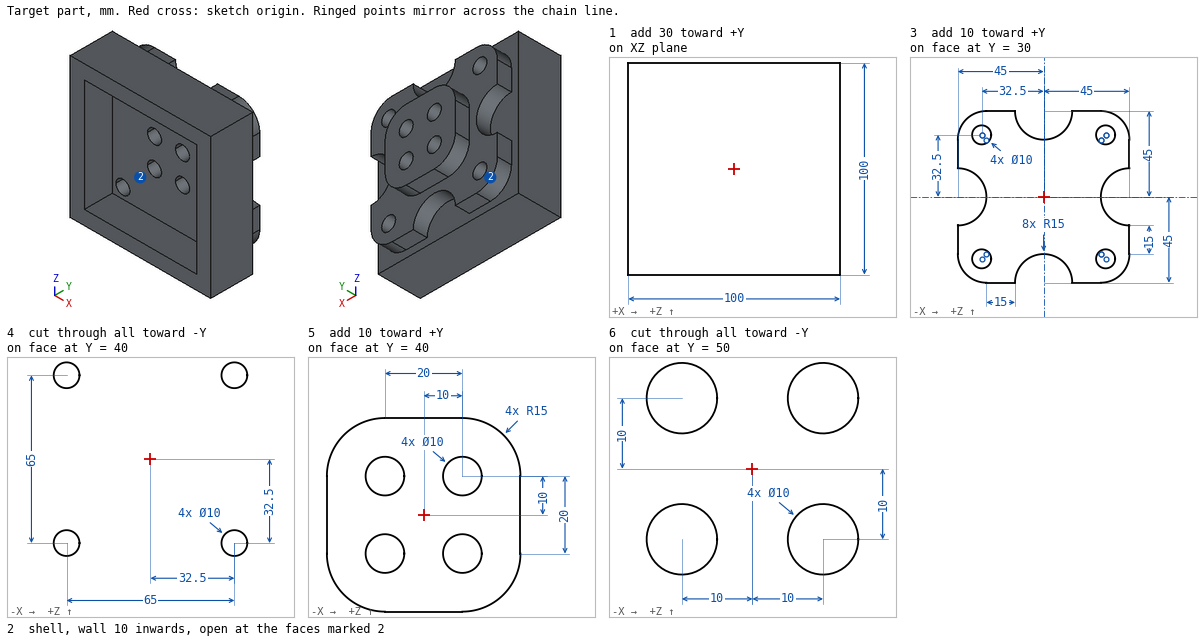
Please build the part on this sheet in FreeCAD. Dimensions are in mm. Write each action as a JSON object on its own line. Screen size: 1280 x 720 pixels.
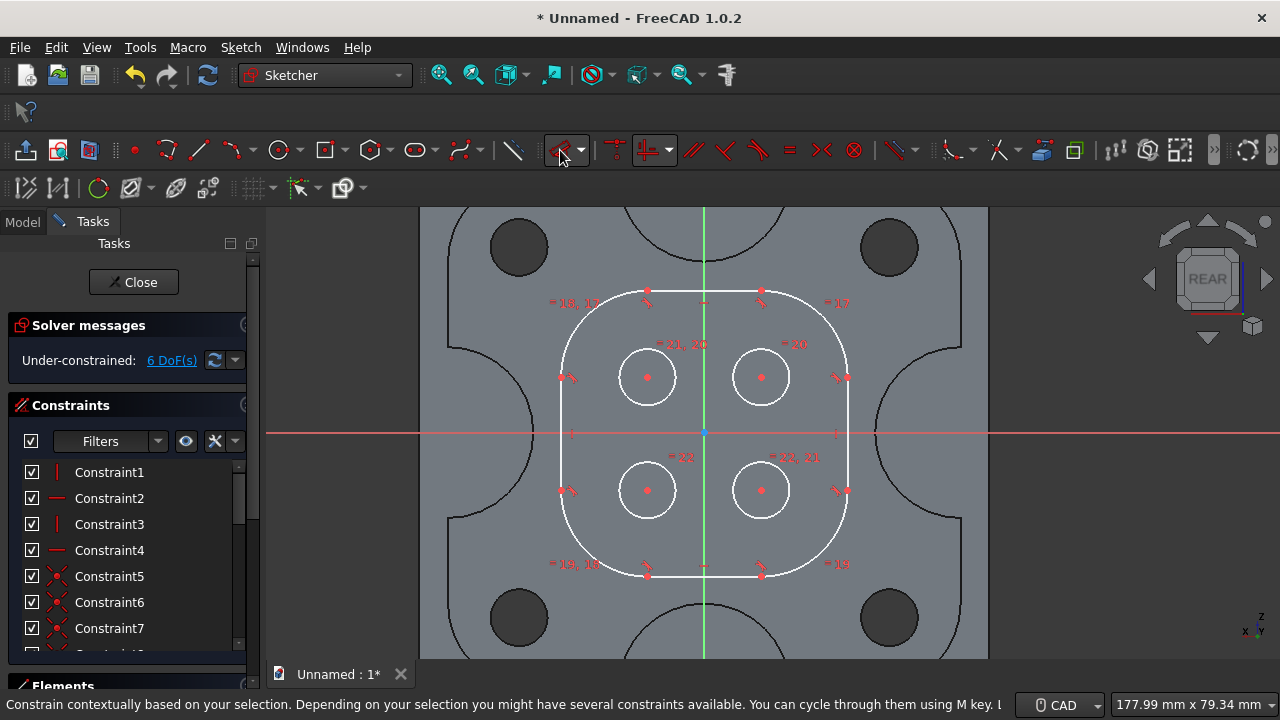
{"action": "left_click", "coordinate": [838, 338]}
{"action": "left_click", "coordinate": [866, 323]}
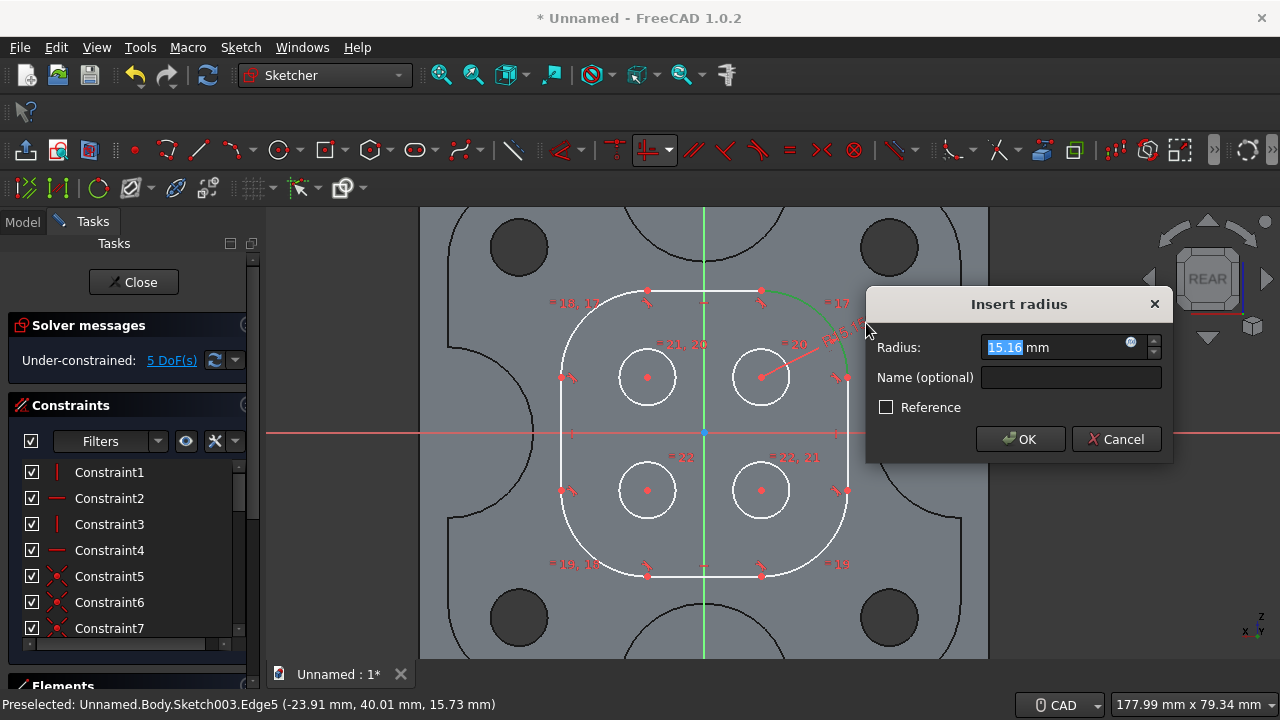
{"action": "type", "text": "15"}
{"action": "key", "text": "Return"}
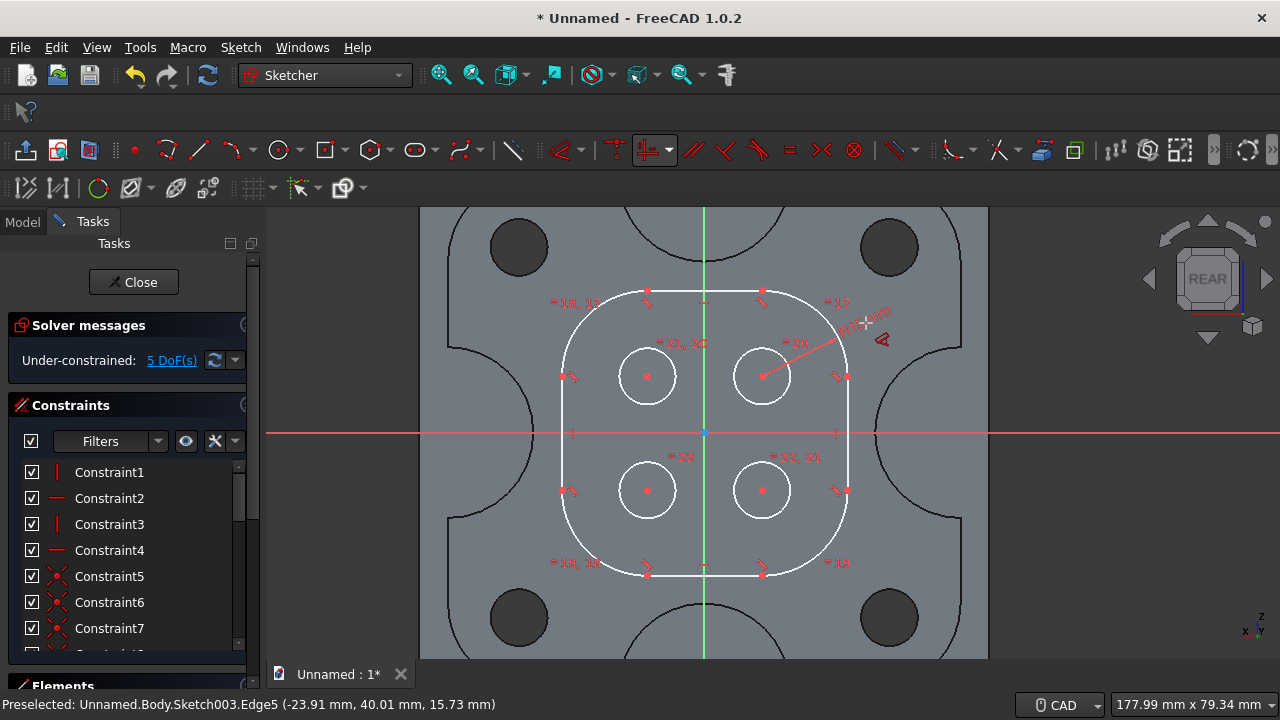
{"action": "left_click", "coordinate": [782, 356]}
{"action": "left_click", "coordinate": [820, 359]}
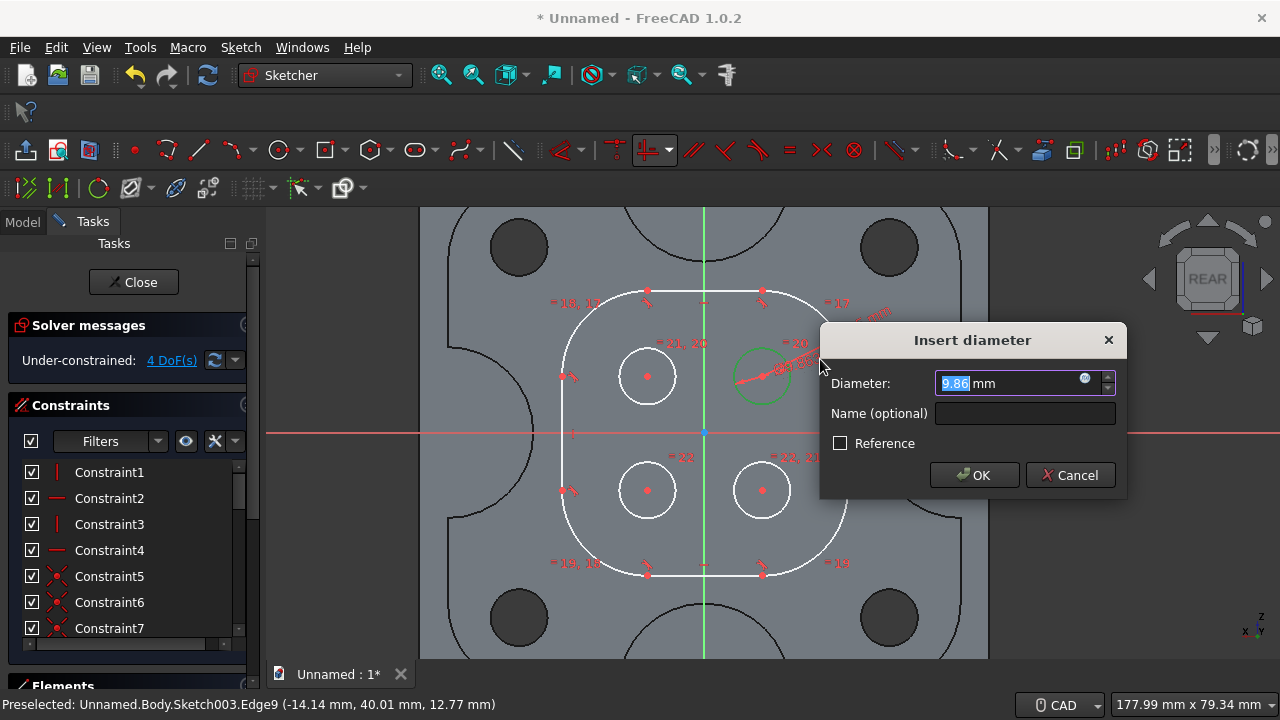
{"action": "type", "text": "10"}
{"action": "key", "text": "Return"}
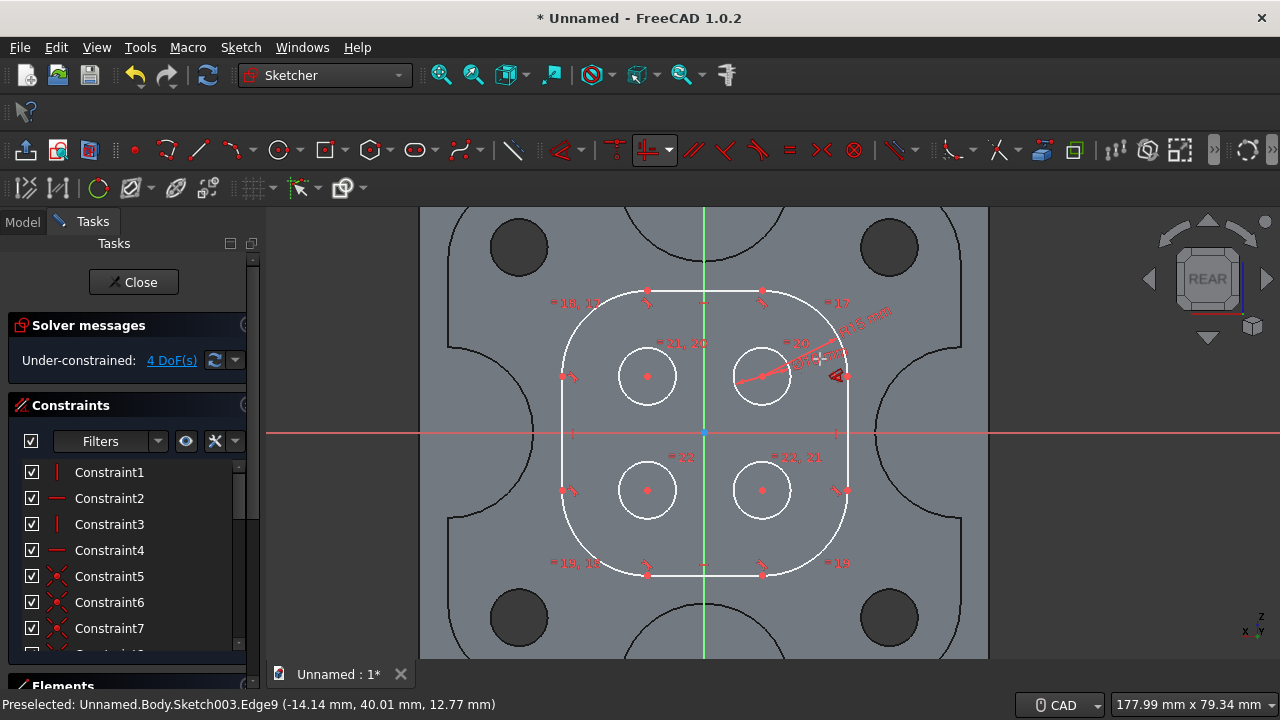
{"action": "left_click", "coordinate": [848, 456]}
{"action": "left_click", "coordinate": [882, 407]}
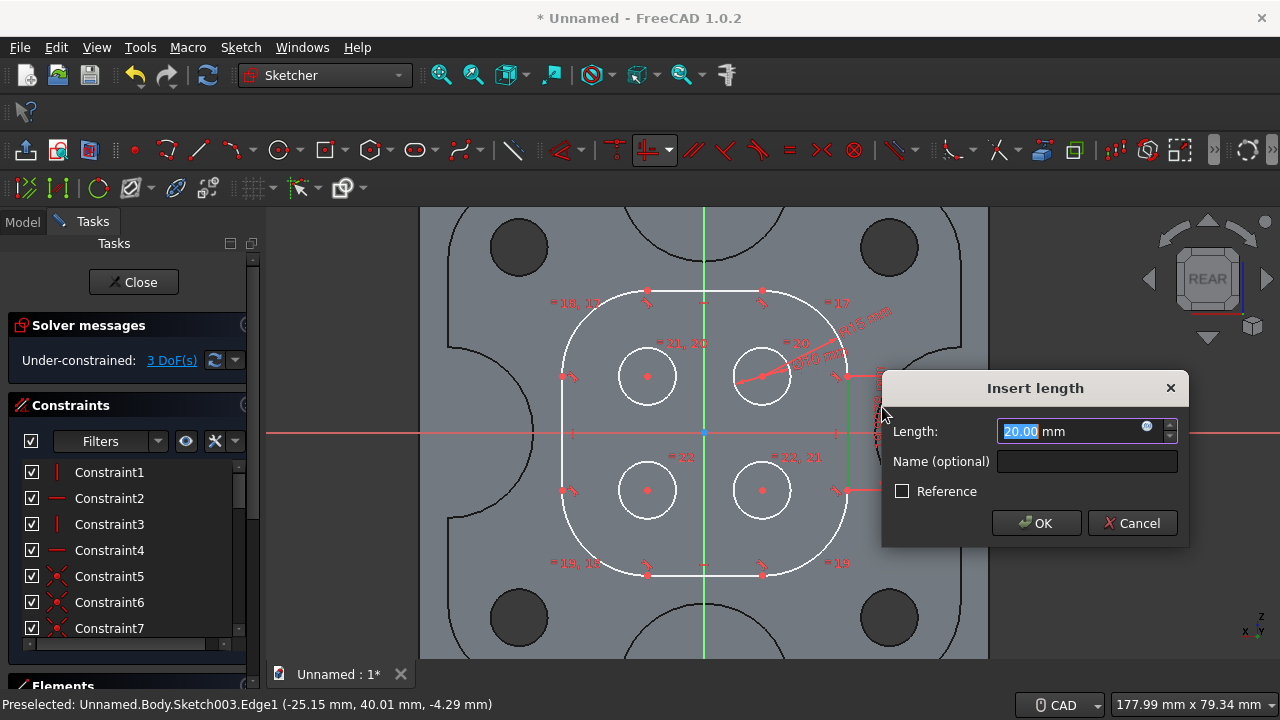
{"action": "type", "text": "20"}
{"action": "key", "text": "Return"}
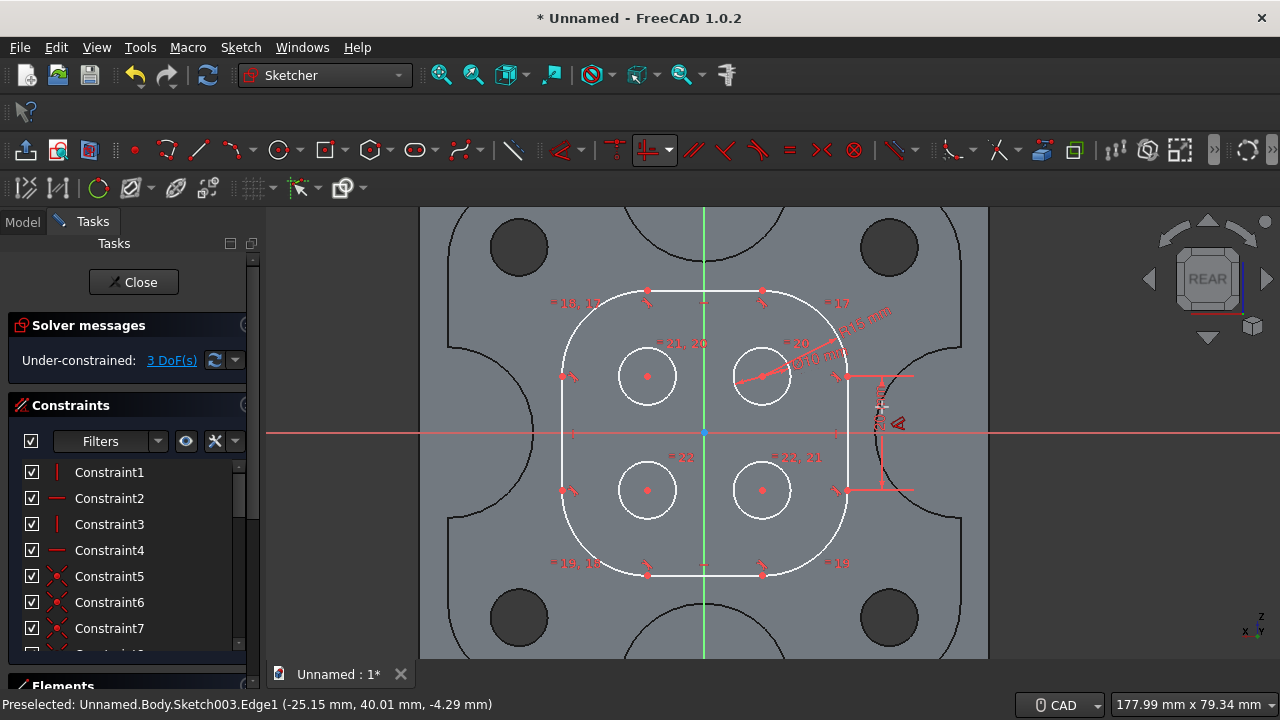
{"action": "left_click", "coordinate": [728, 291]}
{"action": "left_click", "coordinate": [678, 257]}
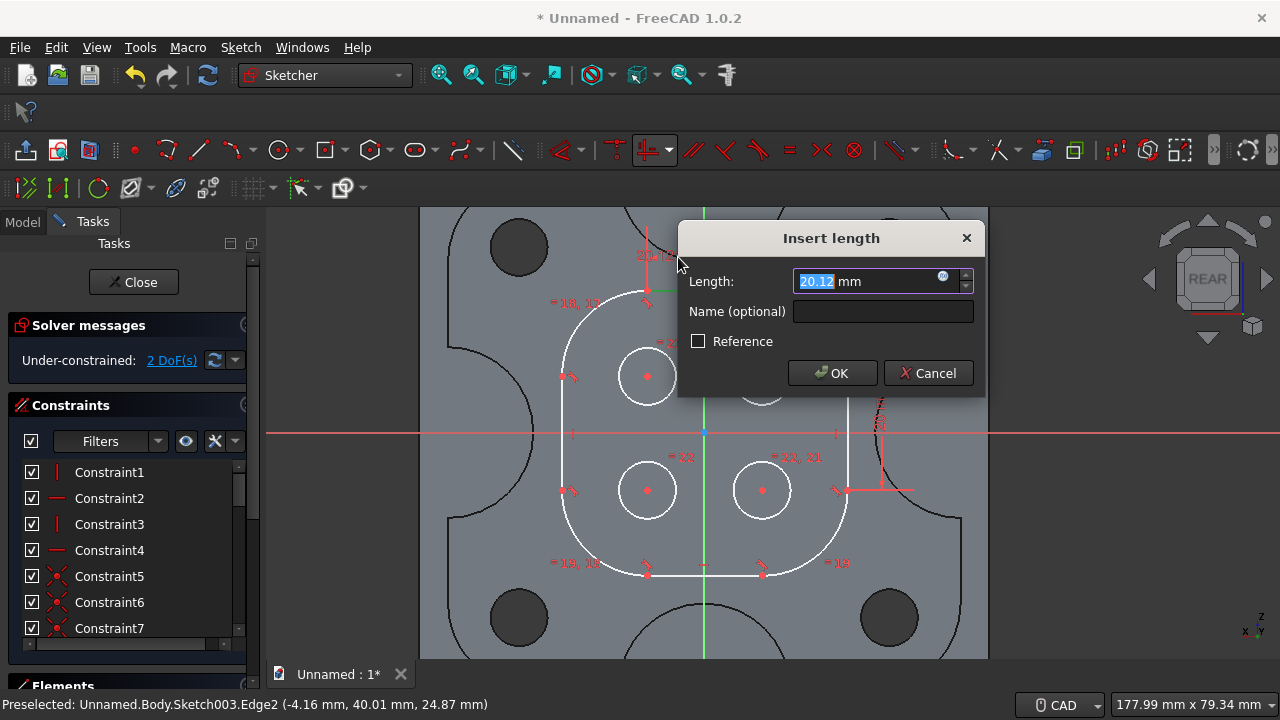
{"action": "type", "text": "20"}
{"action": "key", "text": "Return"}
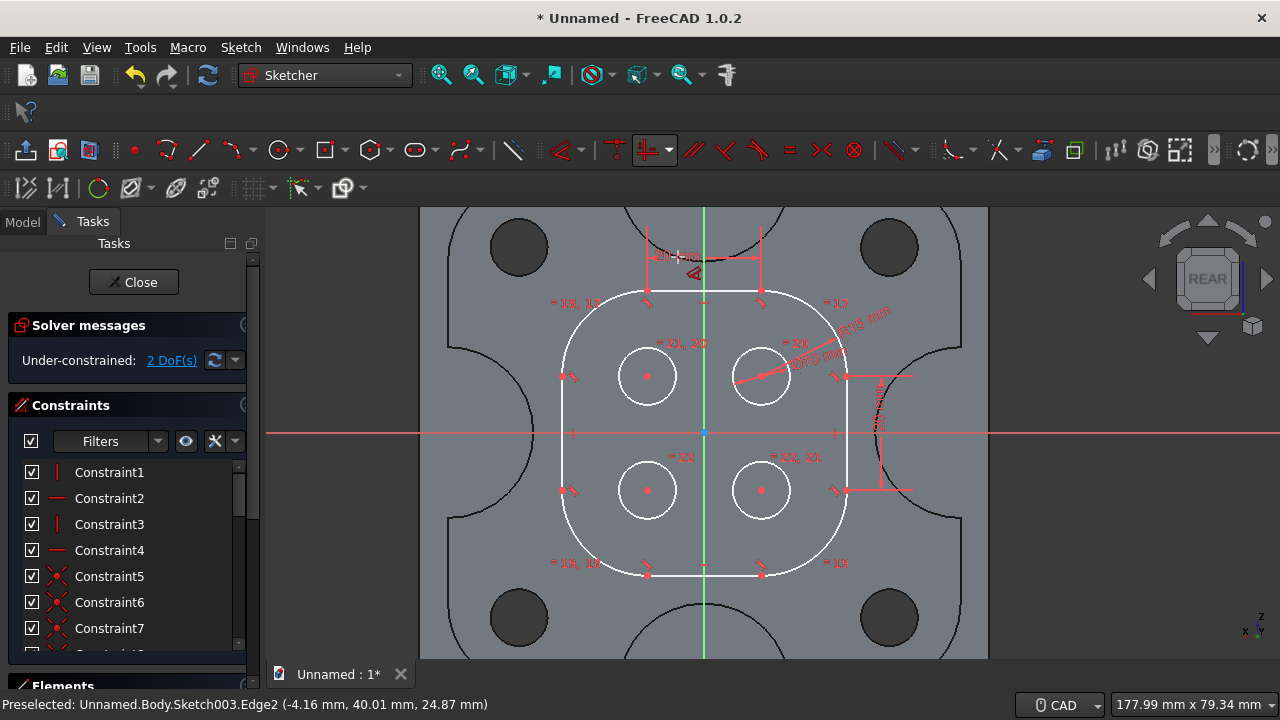
{"action": "left_click", "coordinate": [761, 376]}
{"action": "left_click", "coordinate": [733, 342]}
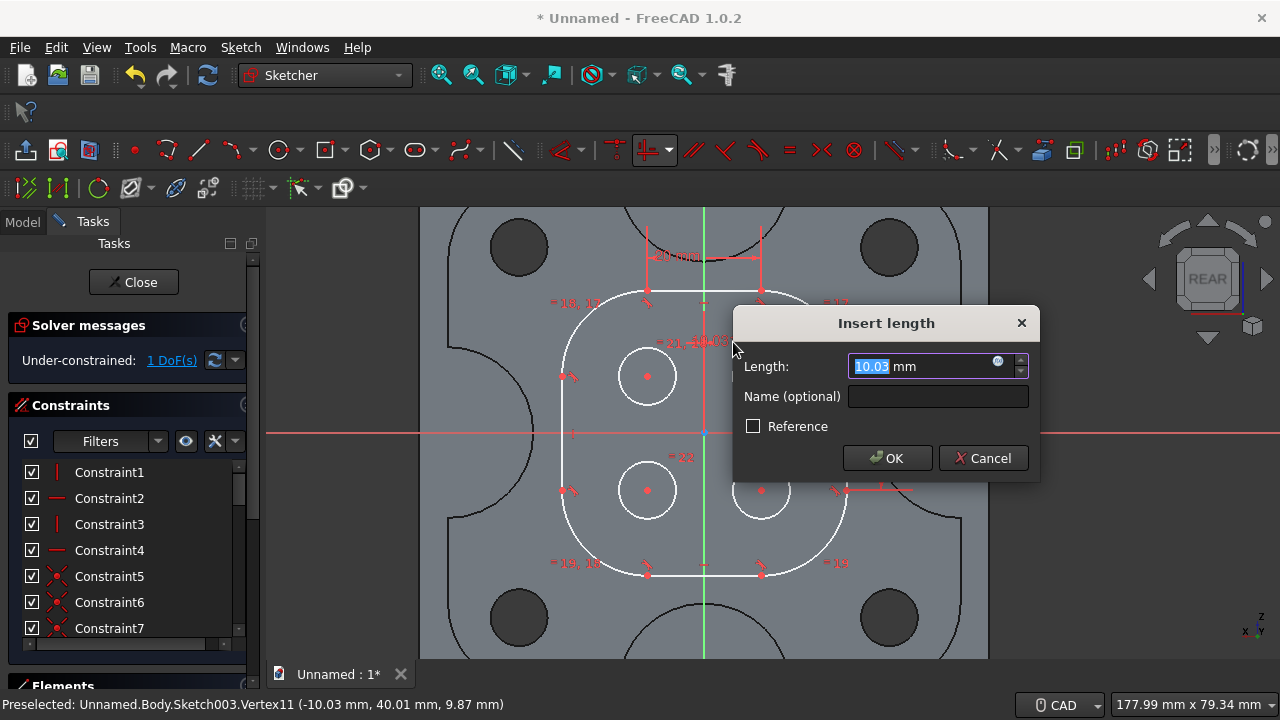
{"action": "type", "text": "10"}
{"action": "key", "text": "Return"}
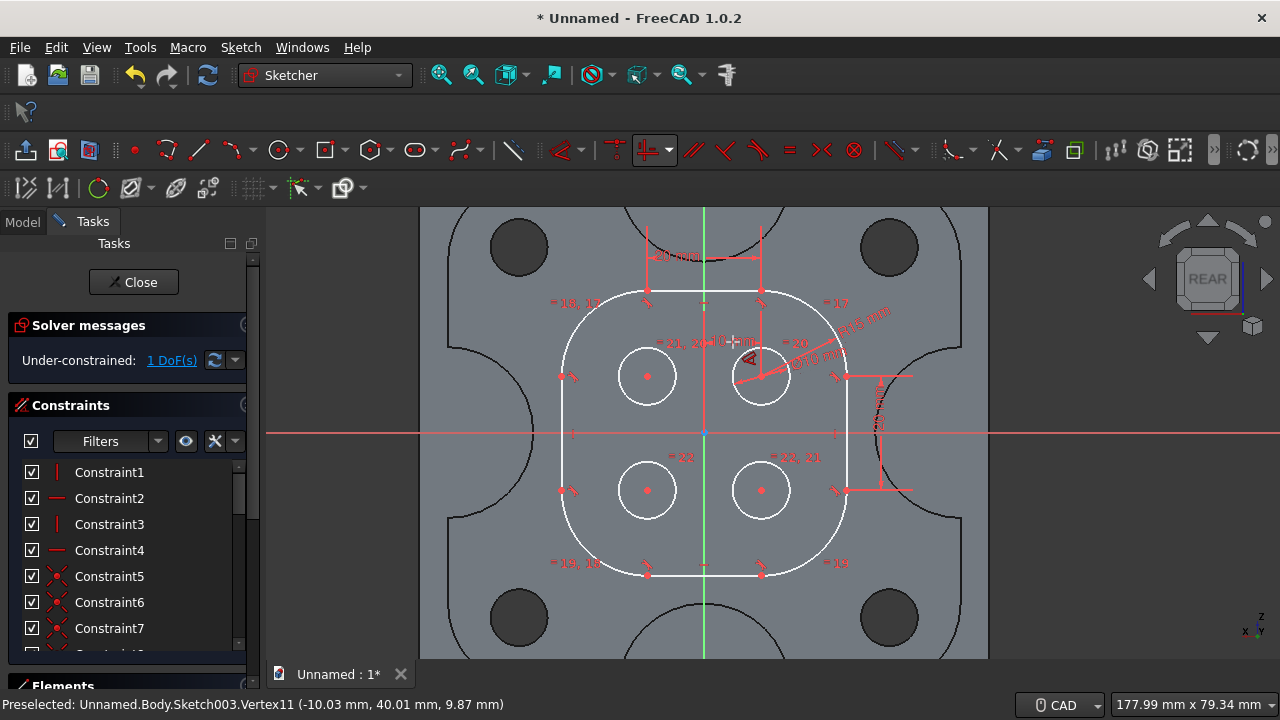
{"action": "left_click", "coordinate": [761, 376]}
{"action": "left_click", "coordinate": [795, 404]}